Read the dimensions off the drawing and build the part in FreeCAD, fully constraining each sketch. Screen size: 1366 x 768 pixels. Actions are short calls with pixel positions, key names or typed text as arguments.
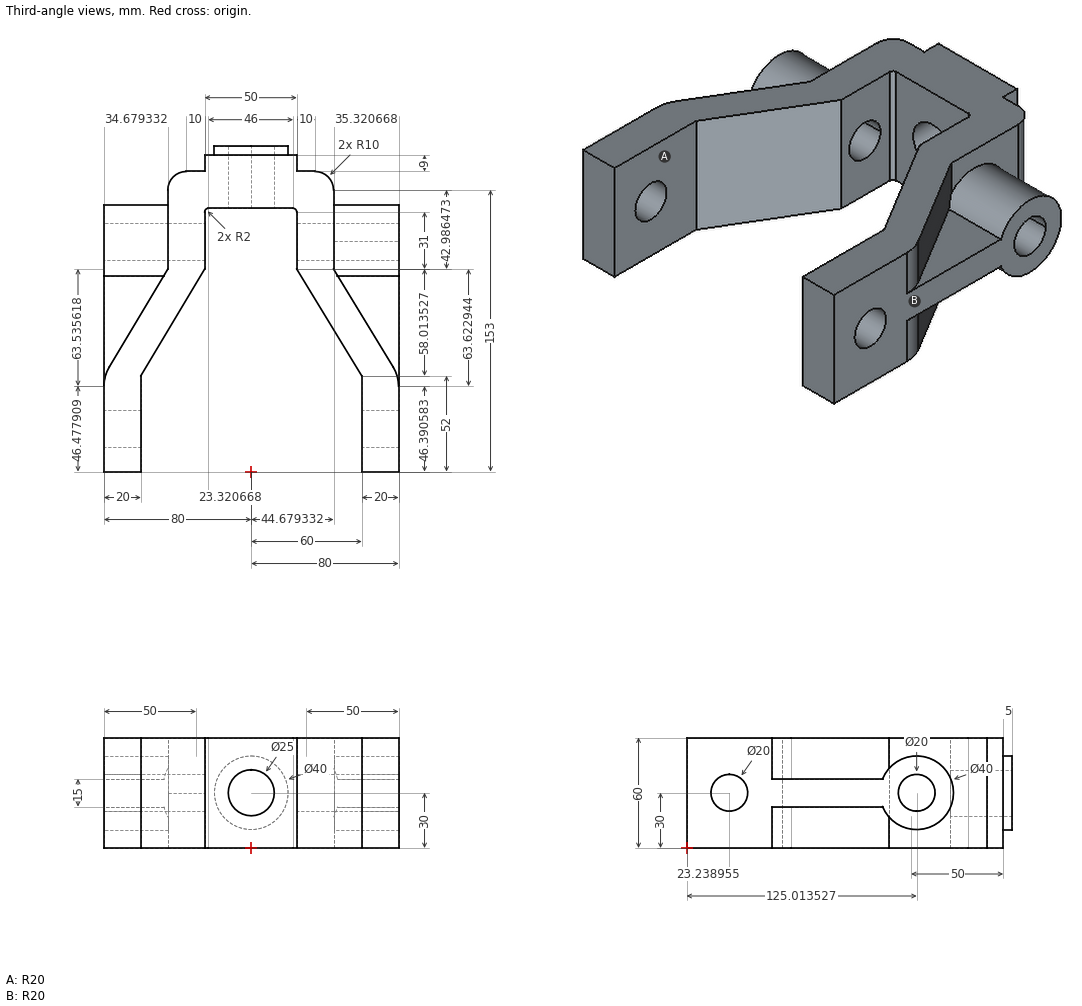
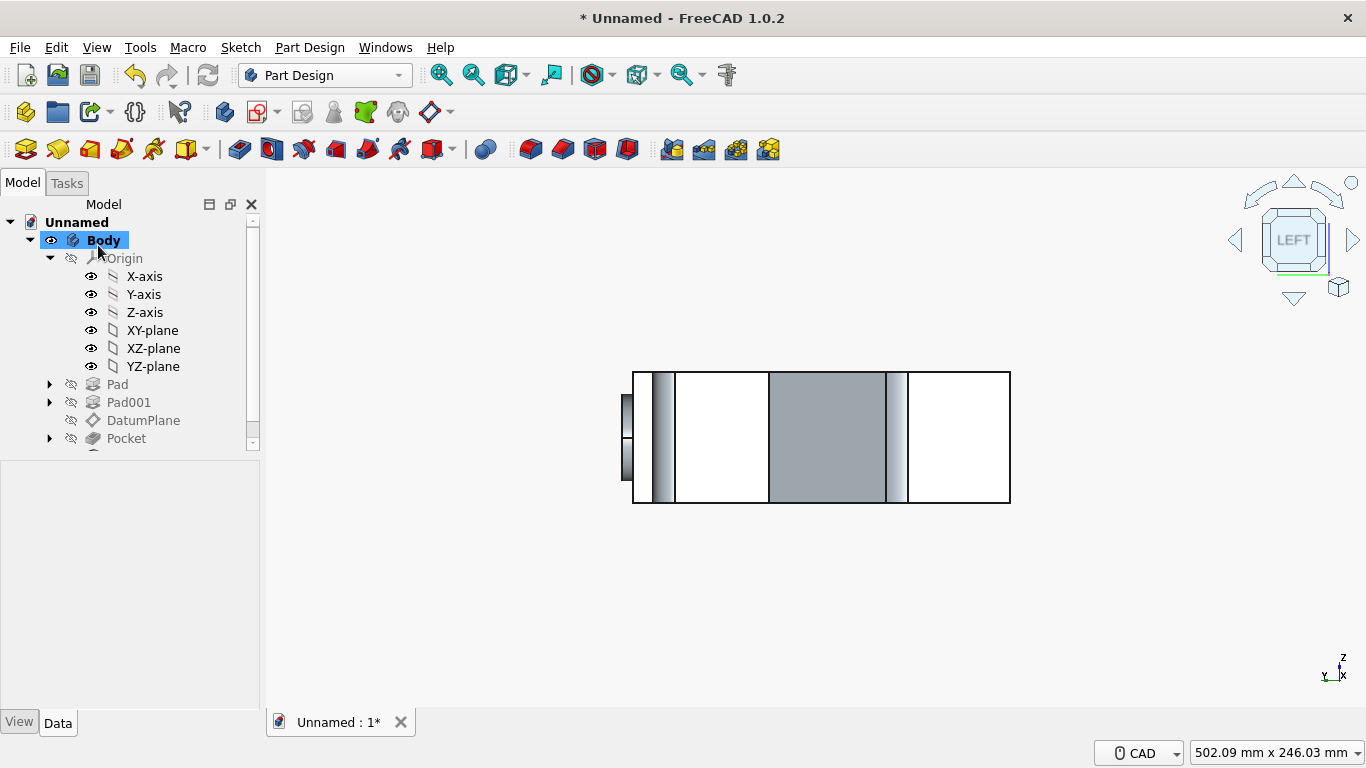
key(0)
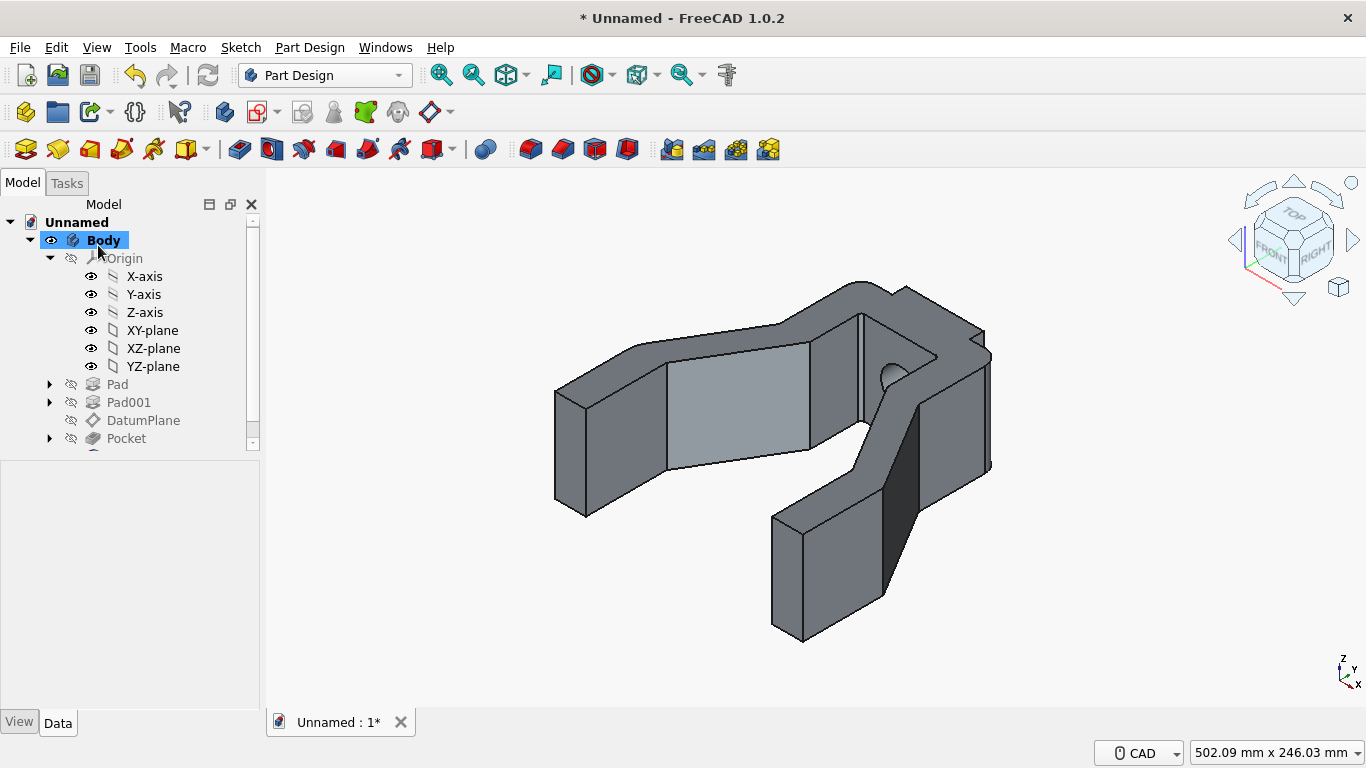
key(2)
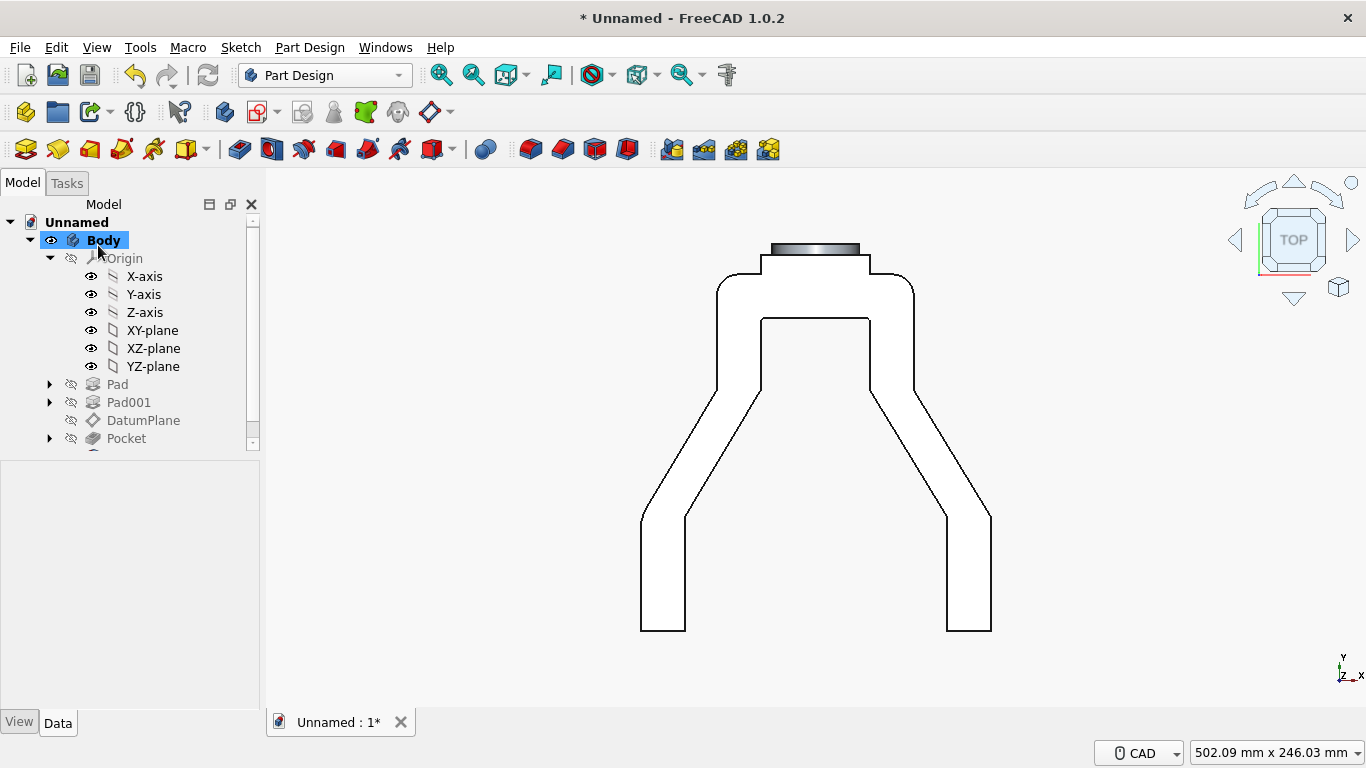
key(1)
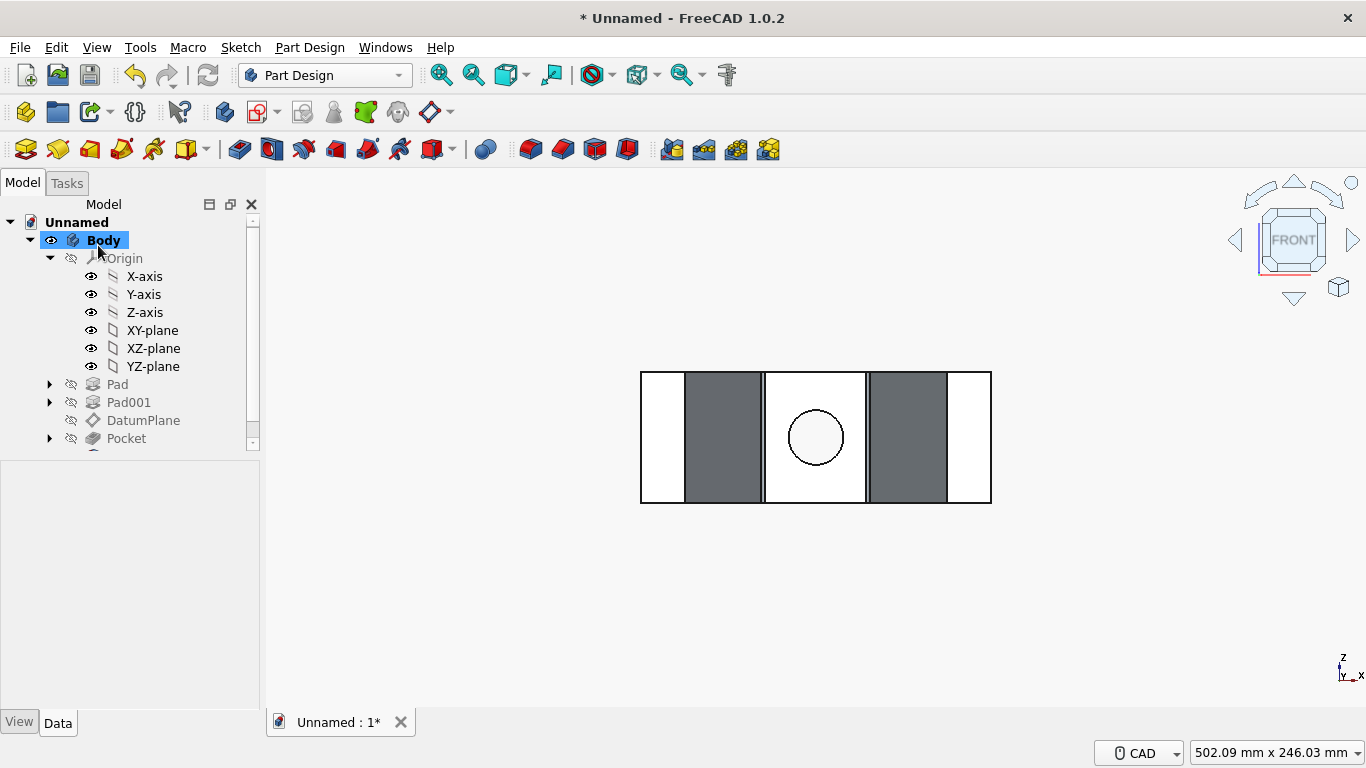
key(v)
key(f)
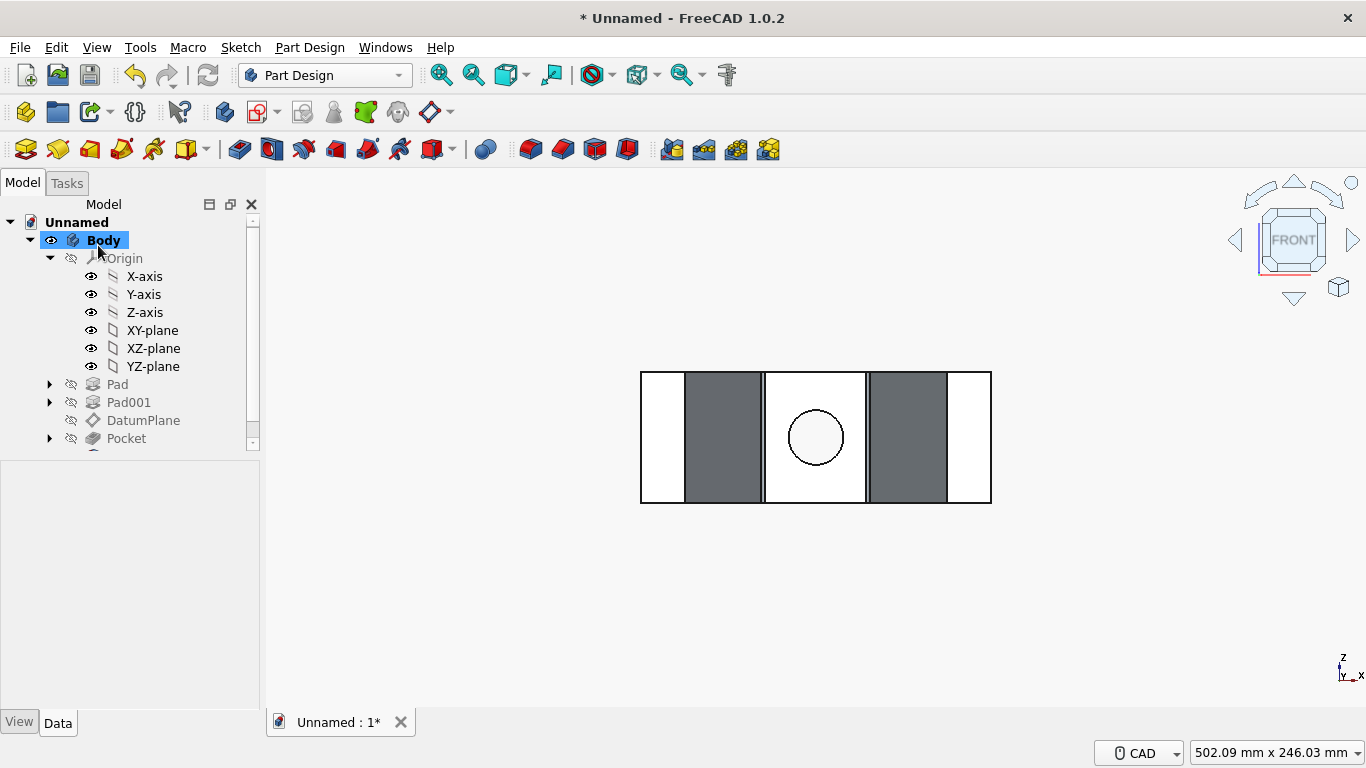
key(3)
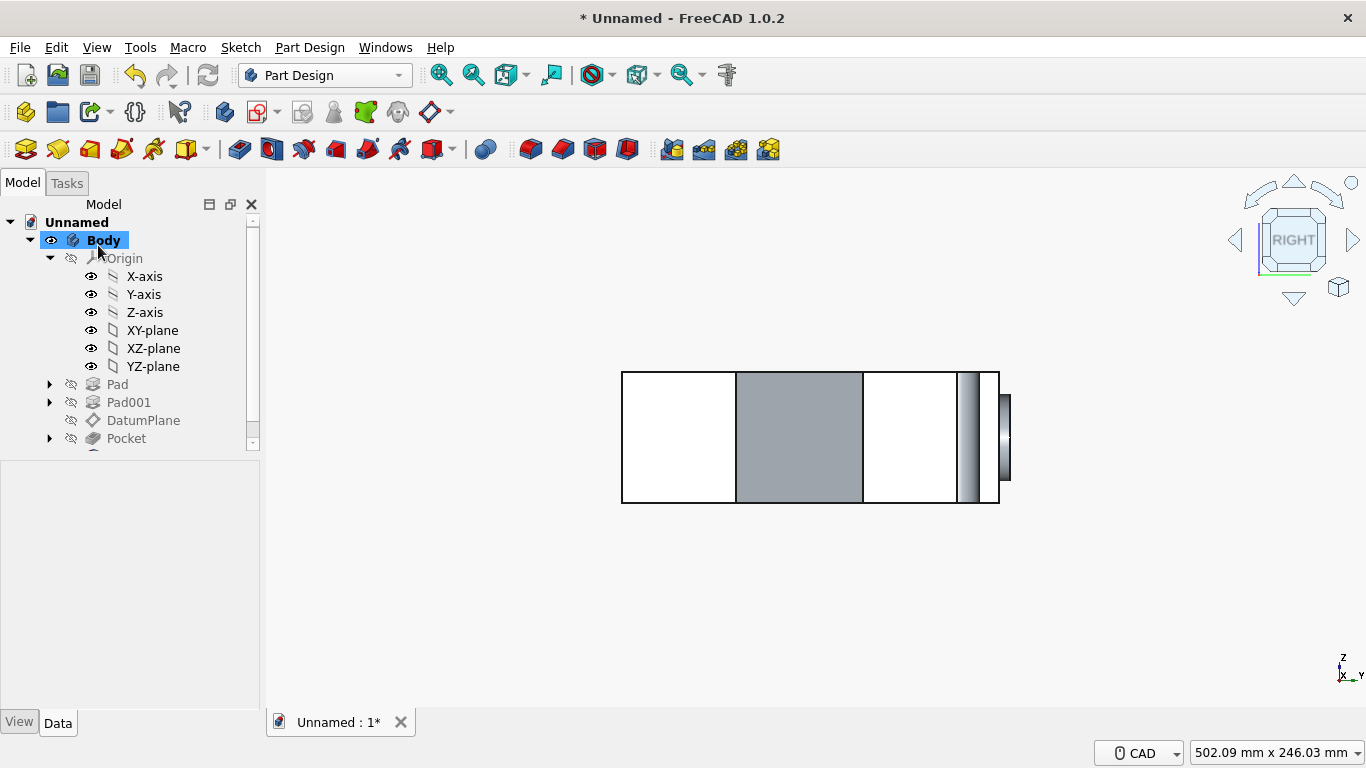
key(v)
key(f)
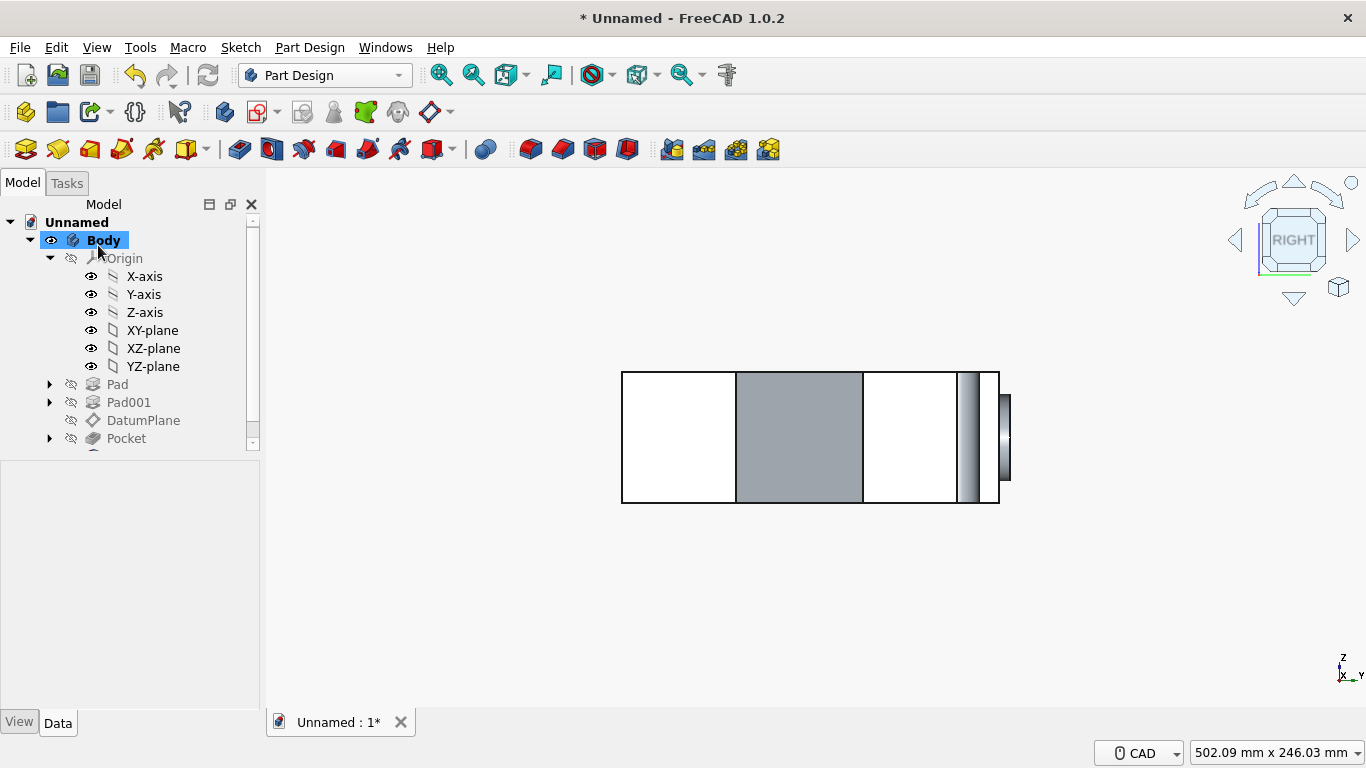
click(736, 436)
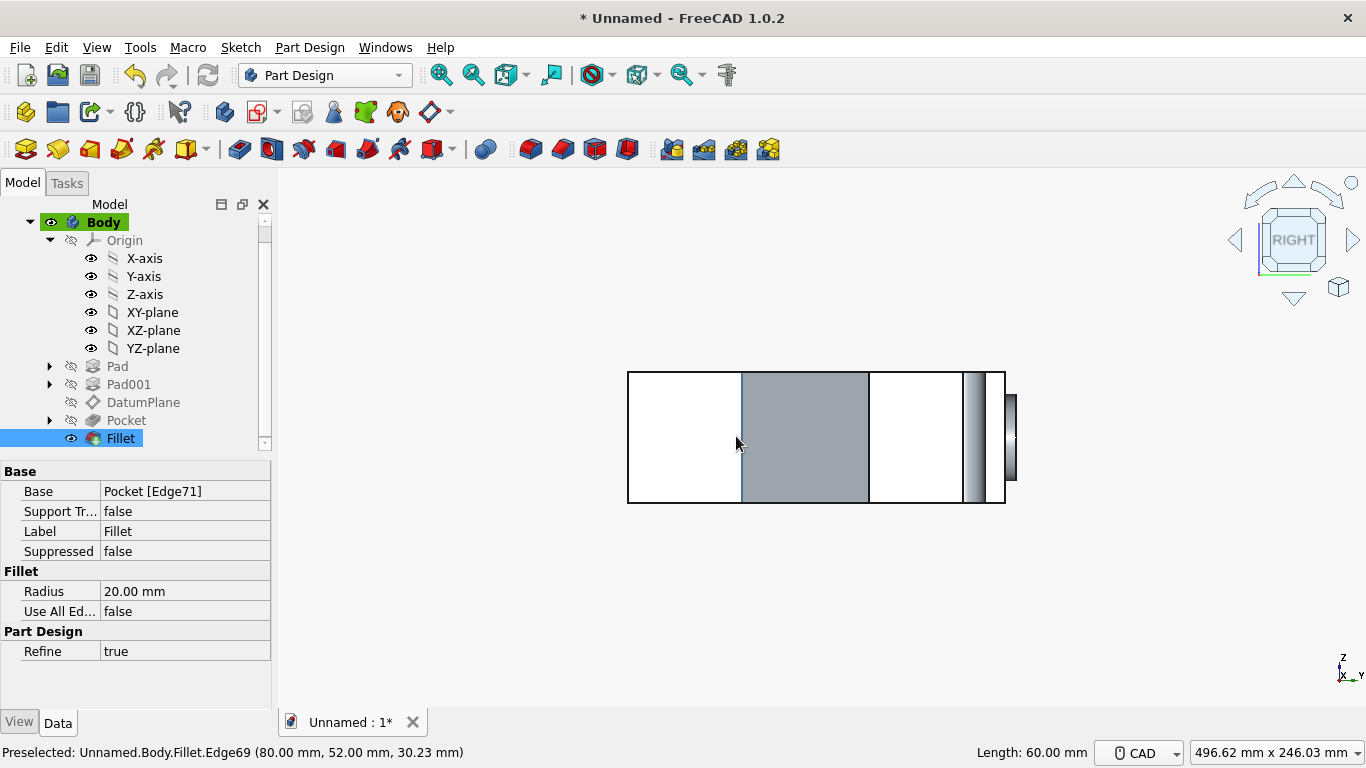
click(532, 150)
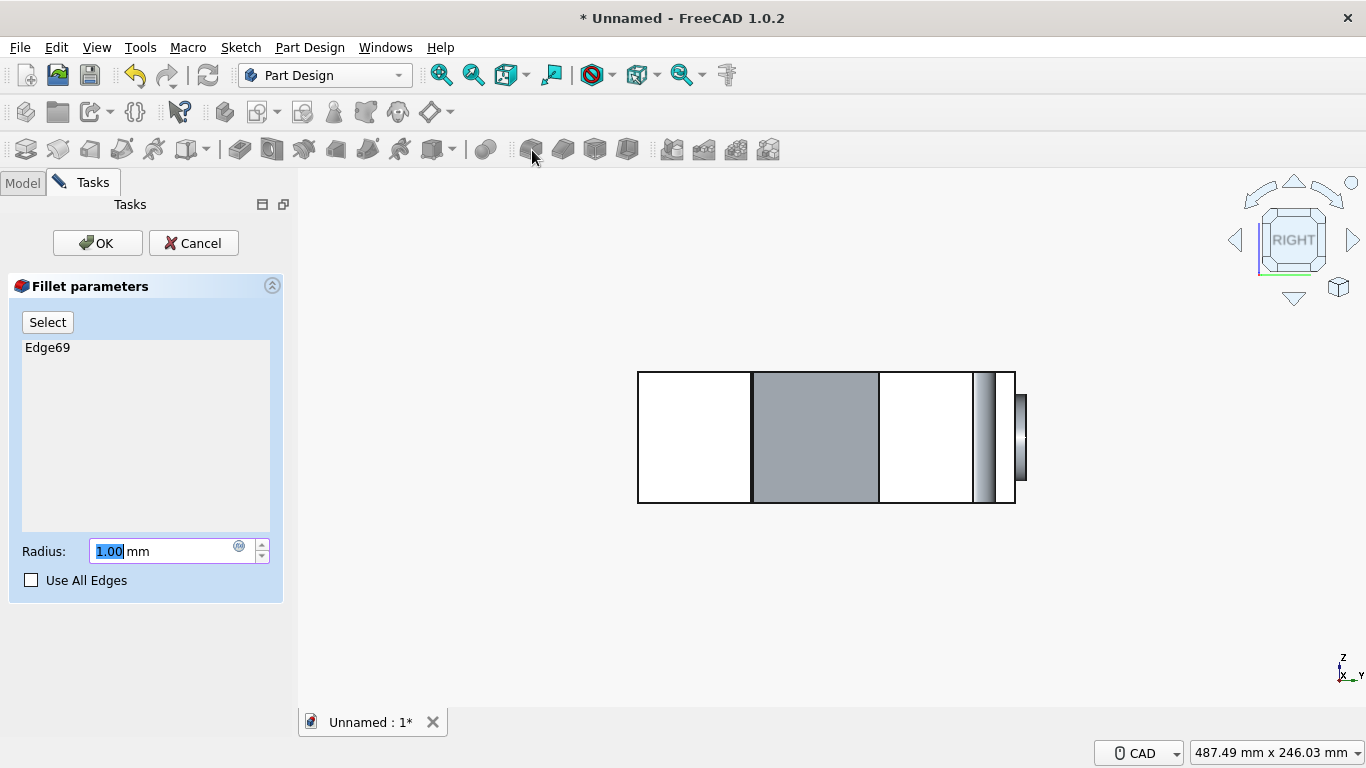
text(20)
key(Tab)